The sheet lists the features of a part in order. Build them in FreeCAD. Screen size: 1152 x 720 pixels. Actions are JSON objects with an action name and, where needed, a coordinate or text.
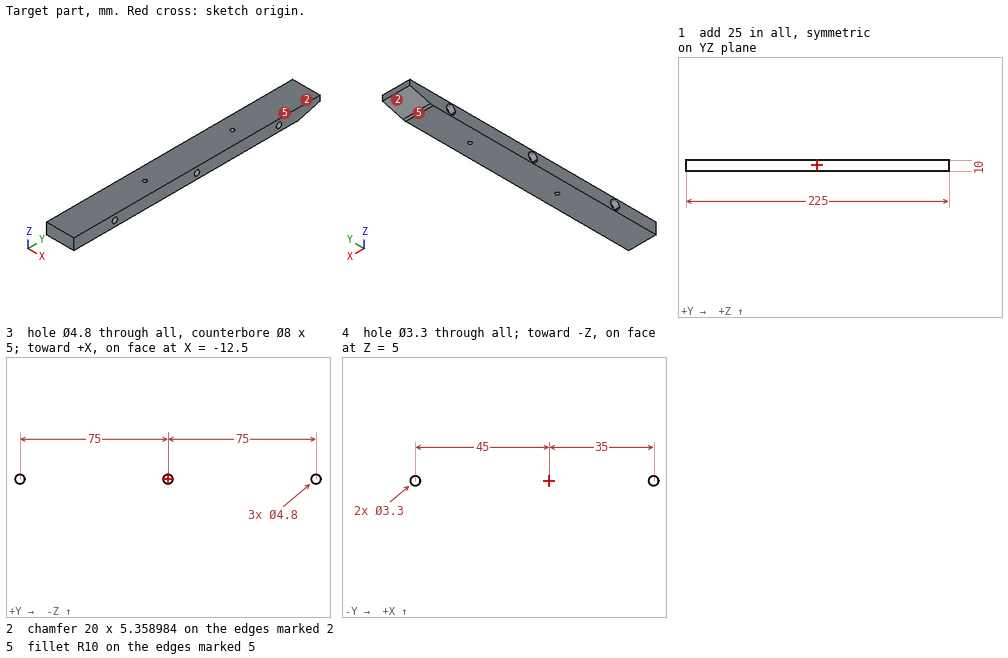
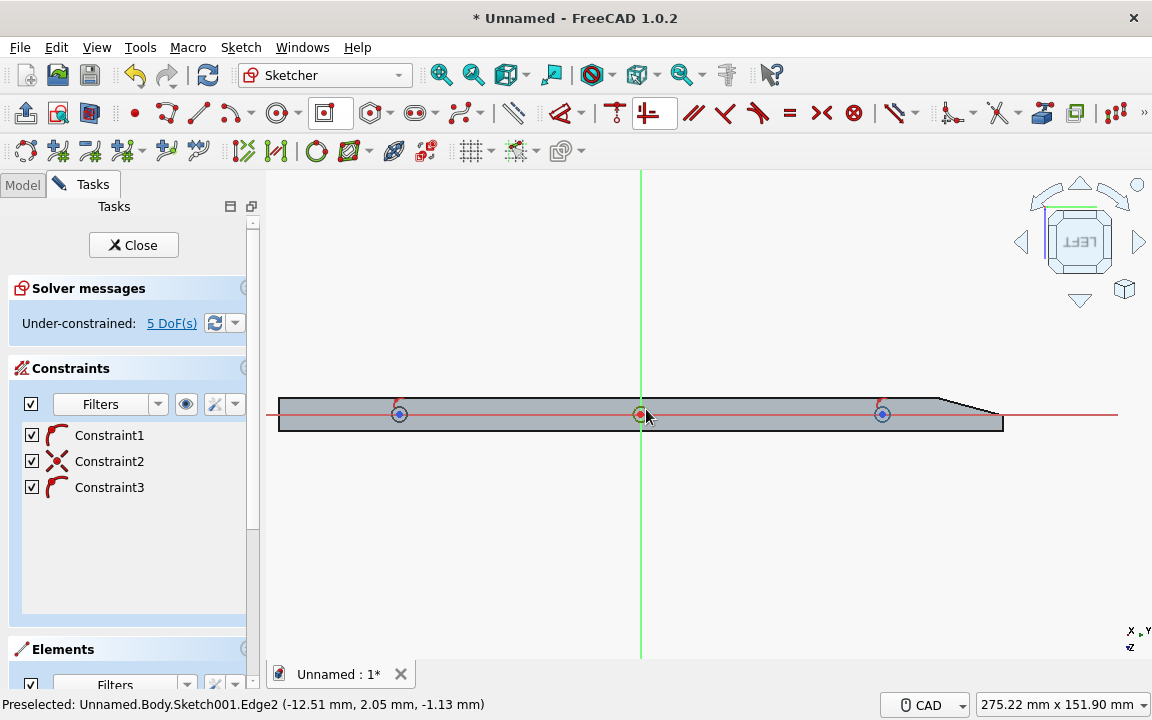
{"action": "scroll", "coordinate": [405, 409], "scroll_direction": "up", "scroll_amount": 5}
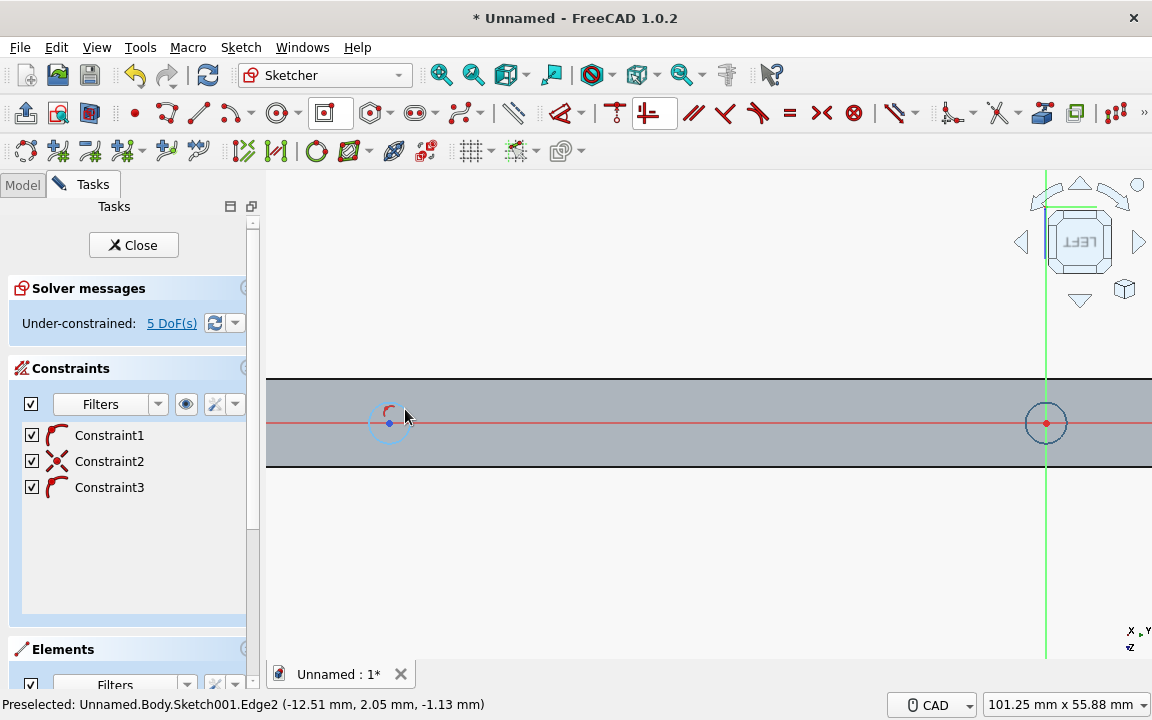
{"action": "left_click", "coordinate": [404, 409]}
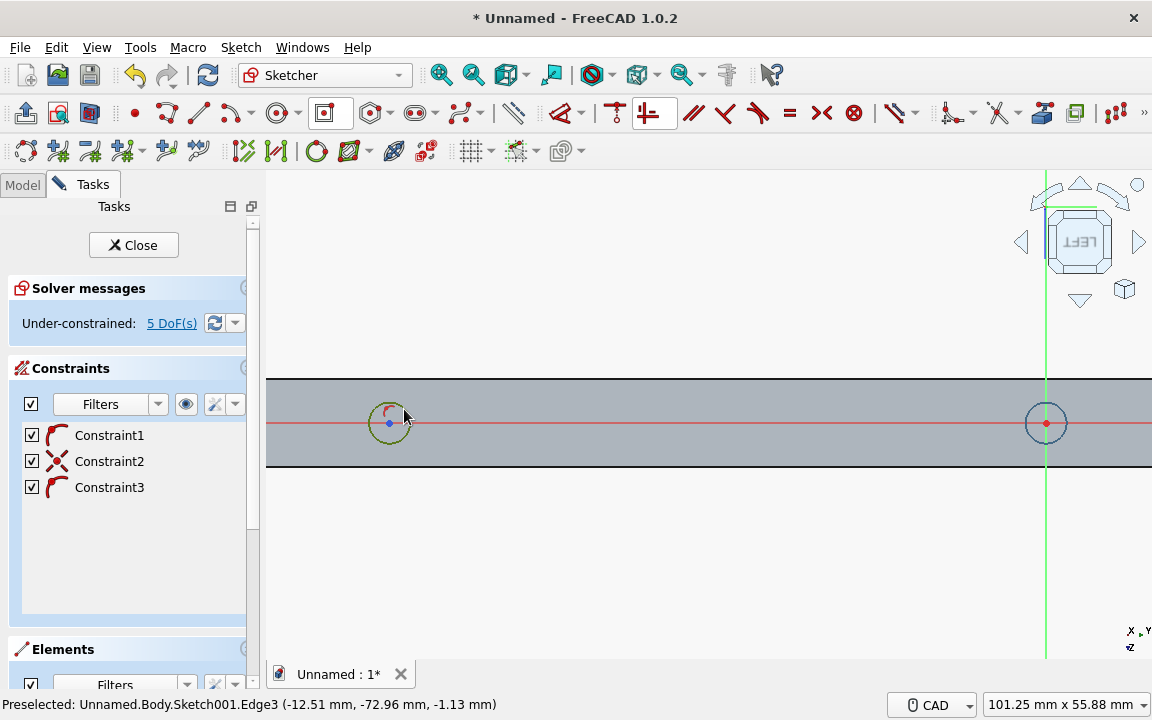
{"action": "left_click", "coordinate": [790, 114]}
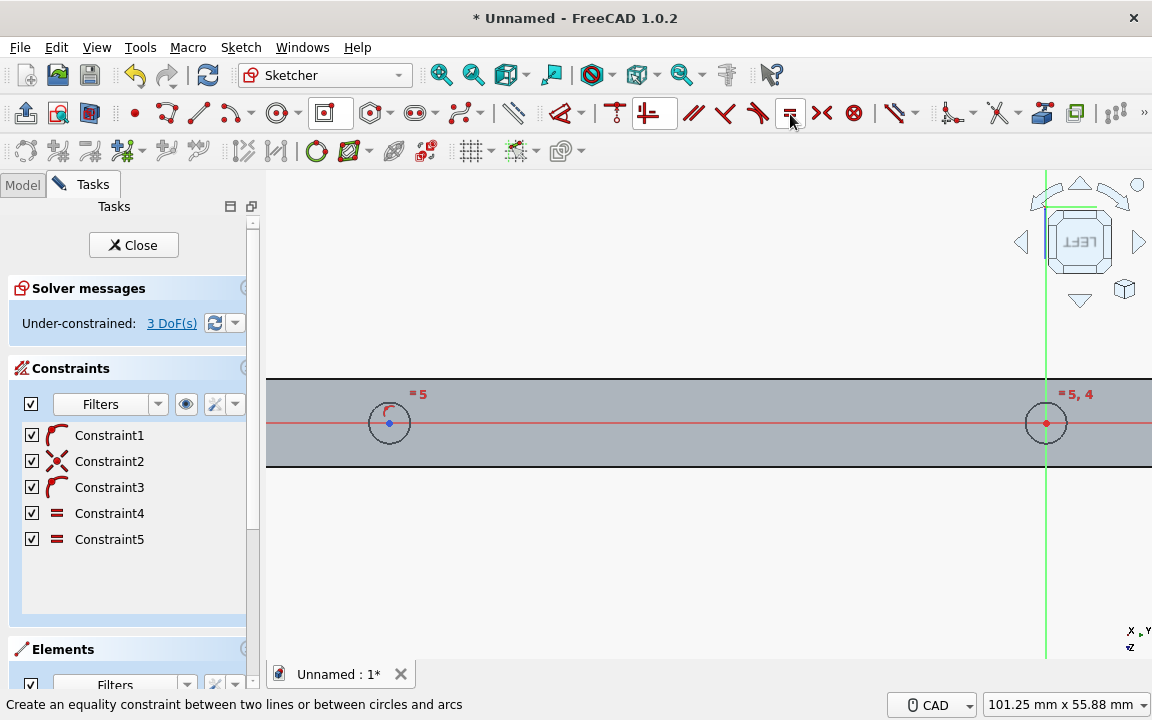
{"action": "key", "text": "d"}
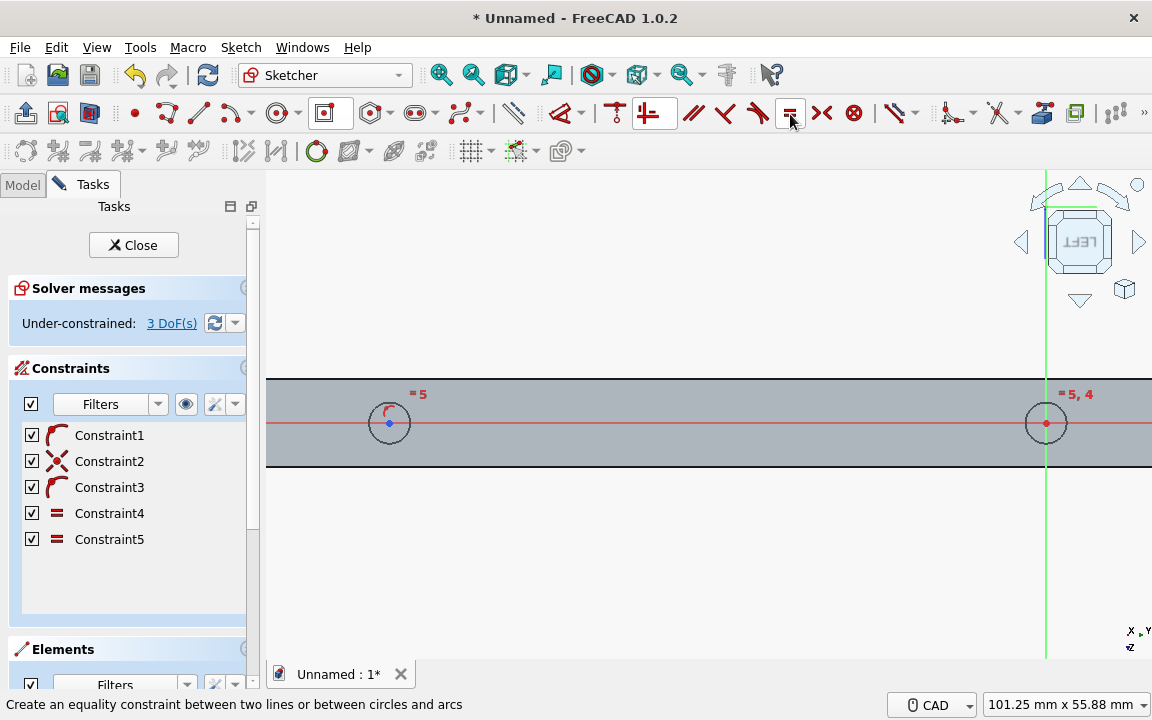
{"action": "scroll", "coordinate": [404, 409], "scroll_direction": "down", "scroll_amount": 5}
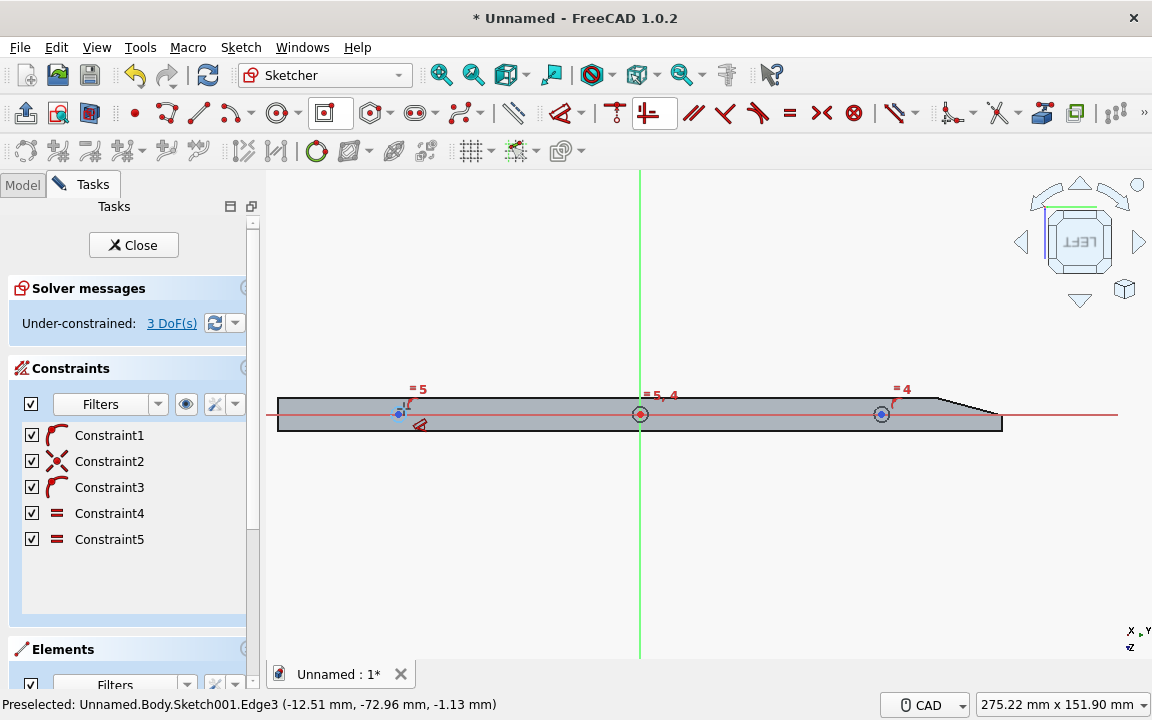
{"action": "scroll", "coordinate": [887, 409], "scroll_direction": "up", "scroll_amount": 5}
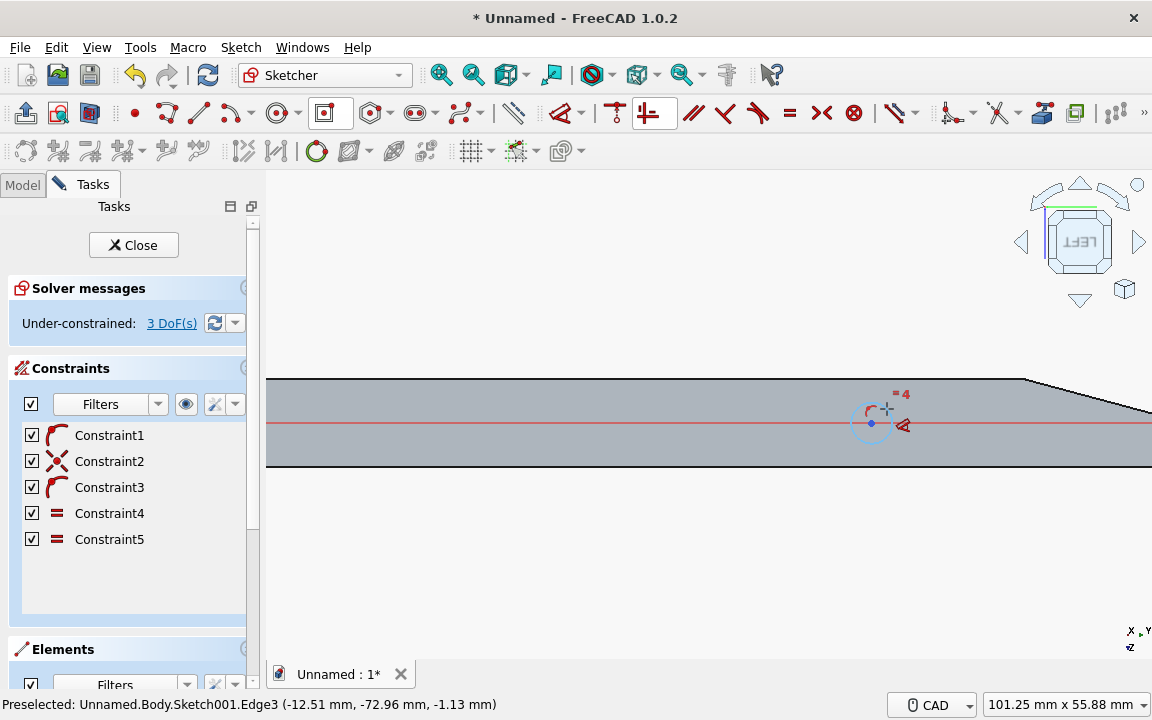
{"action": "left_click", "coordinate": [886, 409]}
{"action": "left_click", "coordinate": [909, 386]}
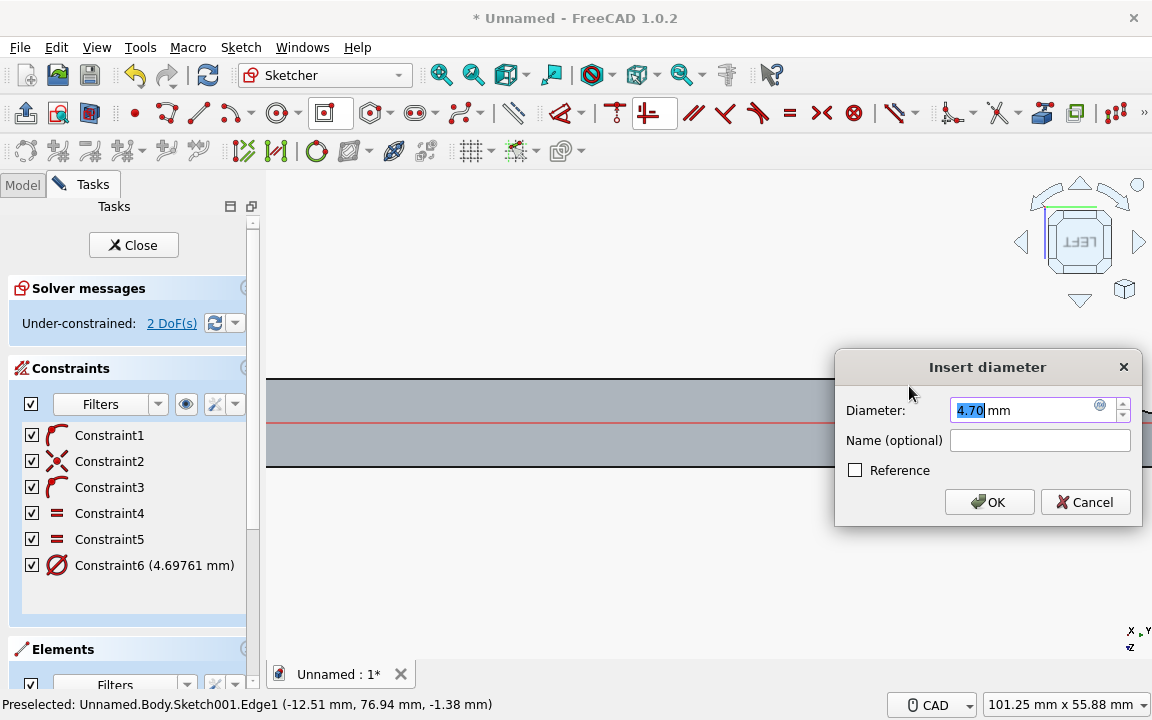
{"action": "type", "text": "4.8"}
{"action": "key", "text": "Return"}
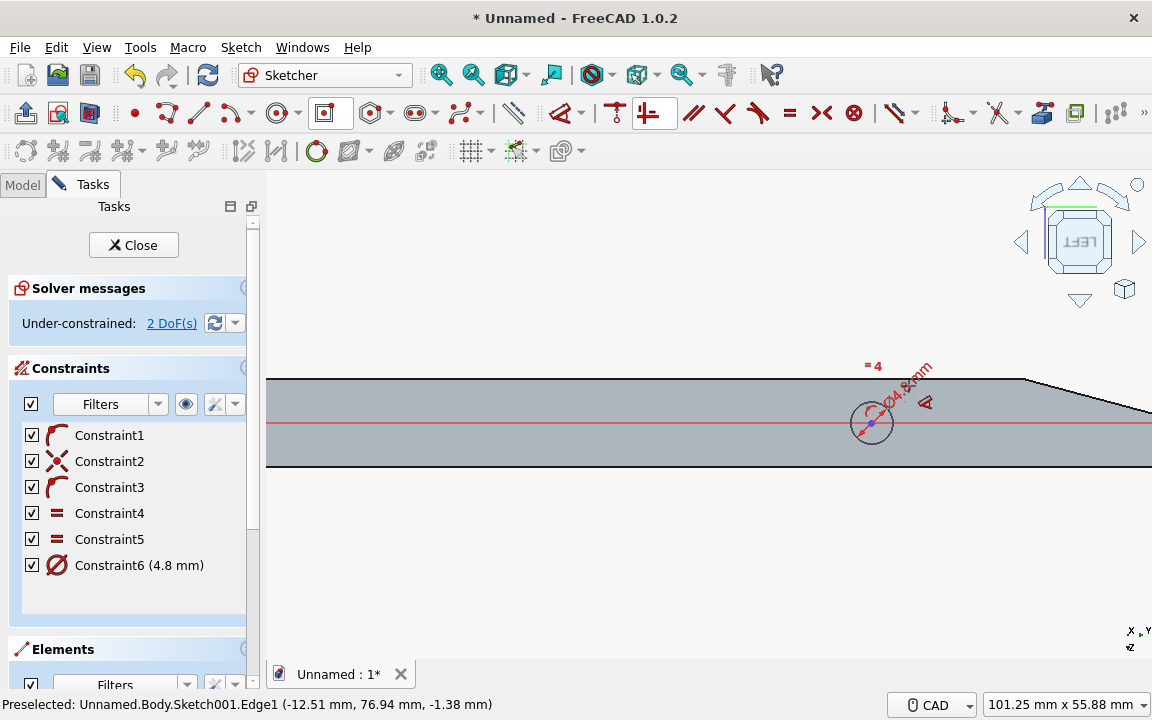
{"action": "left_click", "coordinate": [872, 423]}
{"action": "left_click", "coordinate": [583, 457]}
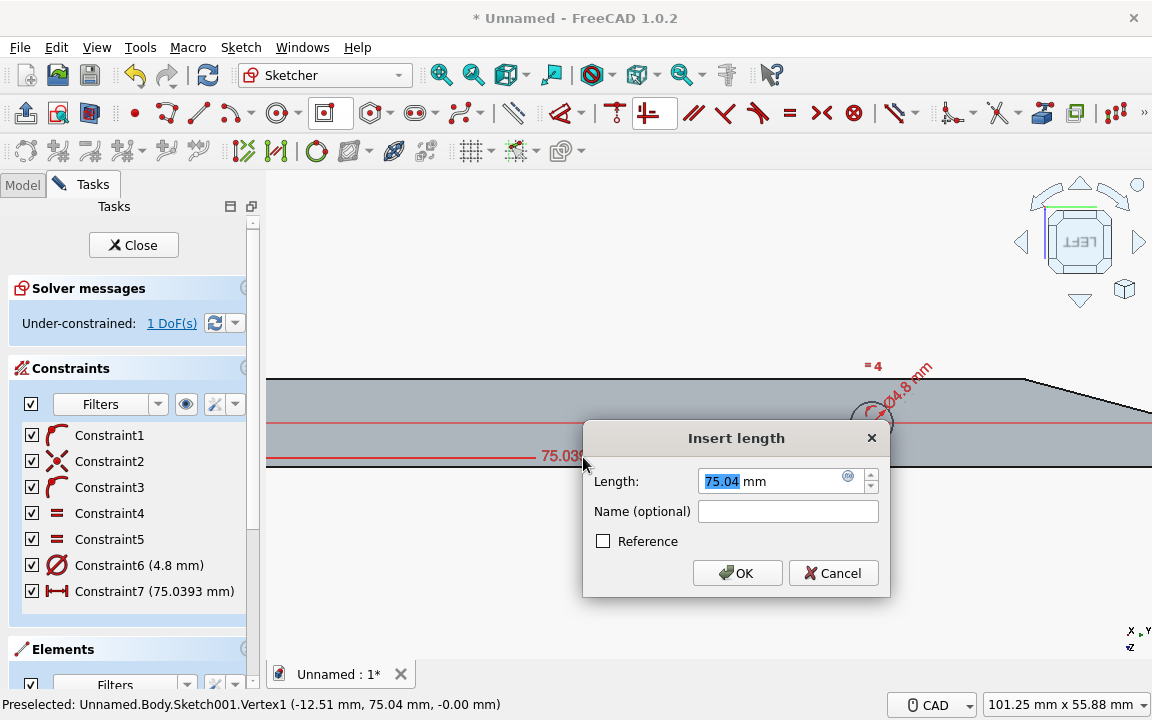
{"action": "type", "text": "75"}
{"action": "key", "text": "Return"}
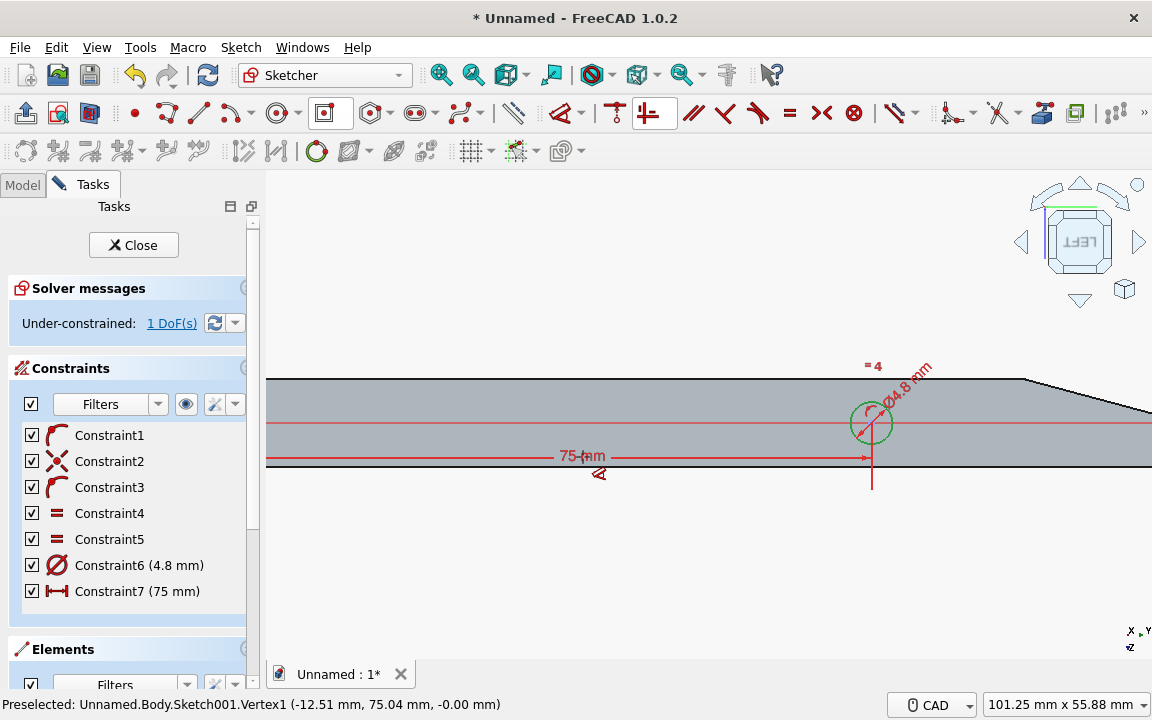
{"action": "scroll", "coordinate": [888, 409], "scroll_direction": "down", "scroll_amount": 5}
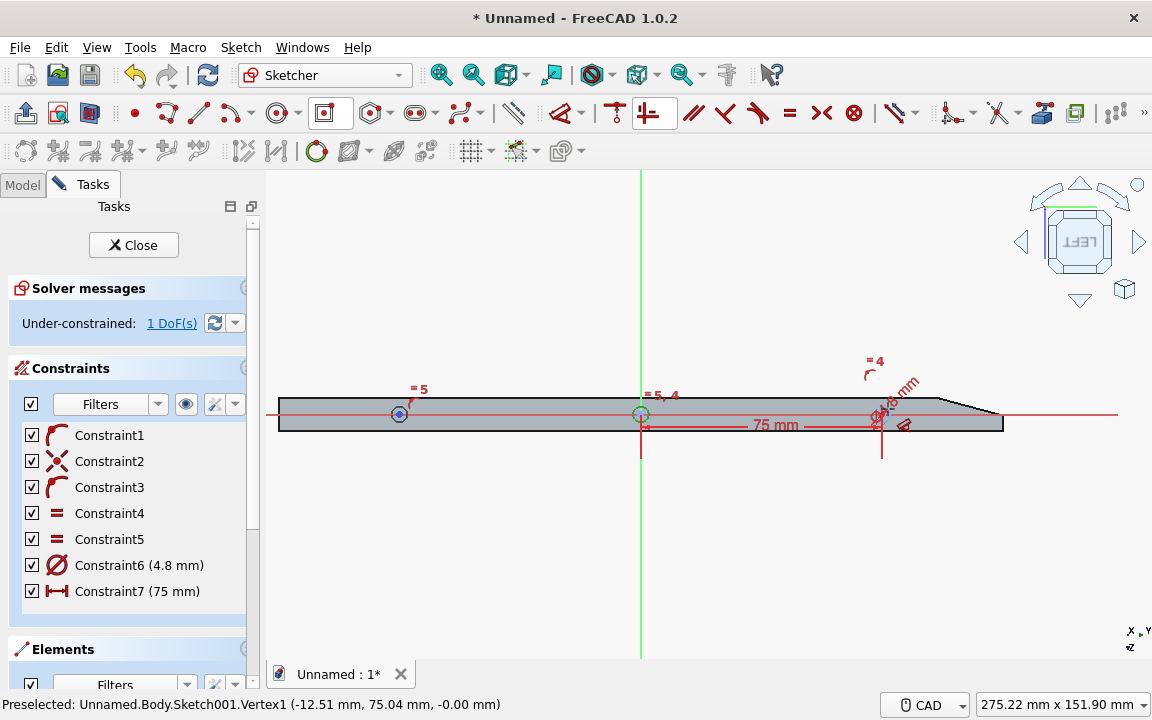
{"action": "left_click", "coordinate": [399, 414]}
{"action": "left_click", "coordinate": [520, 448]}